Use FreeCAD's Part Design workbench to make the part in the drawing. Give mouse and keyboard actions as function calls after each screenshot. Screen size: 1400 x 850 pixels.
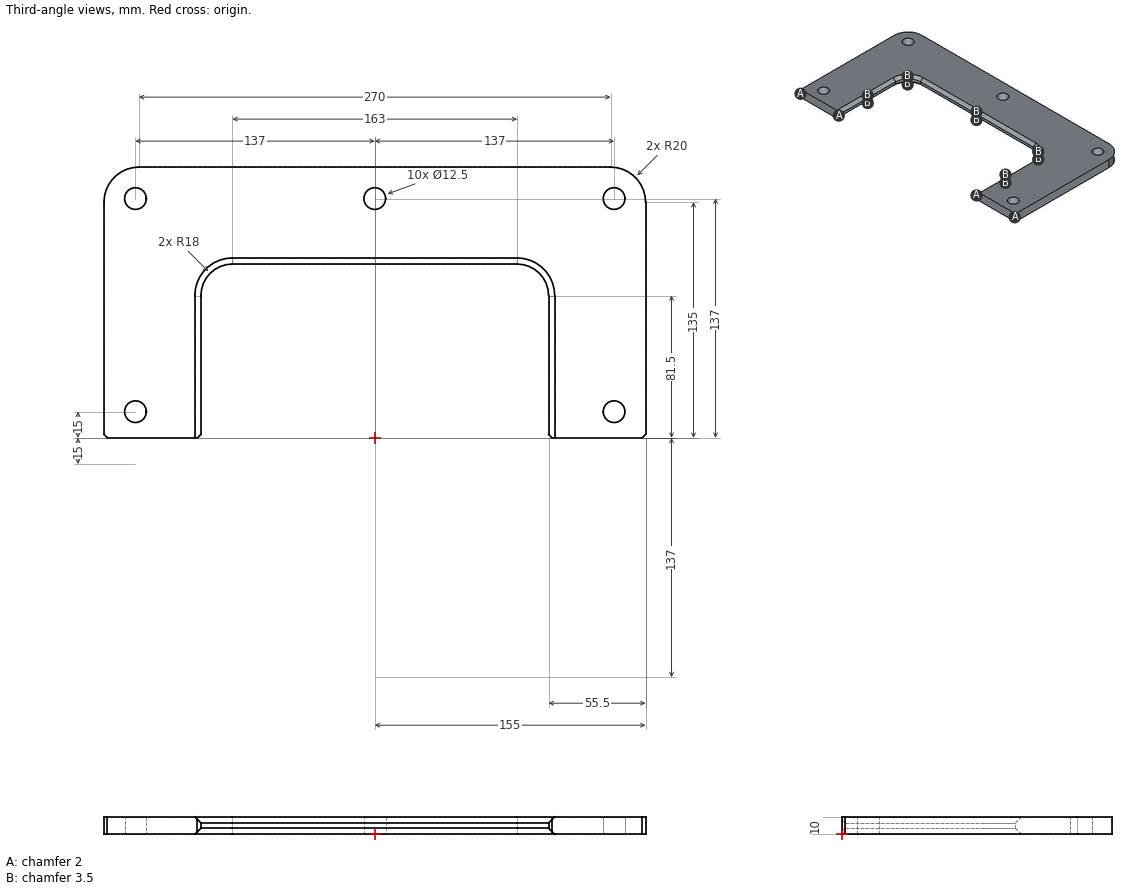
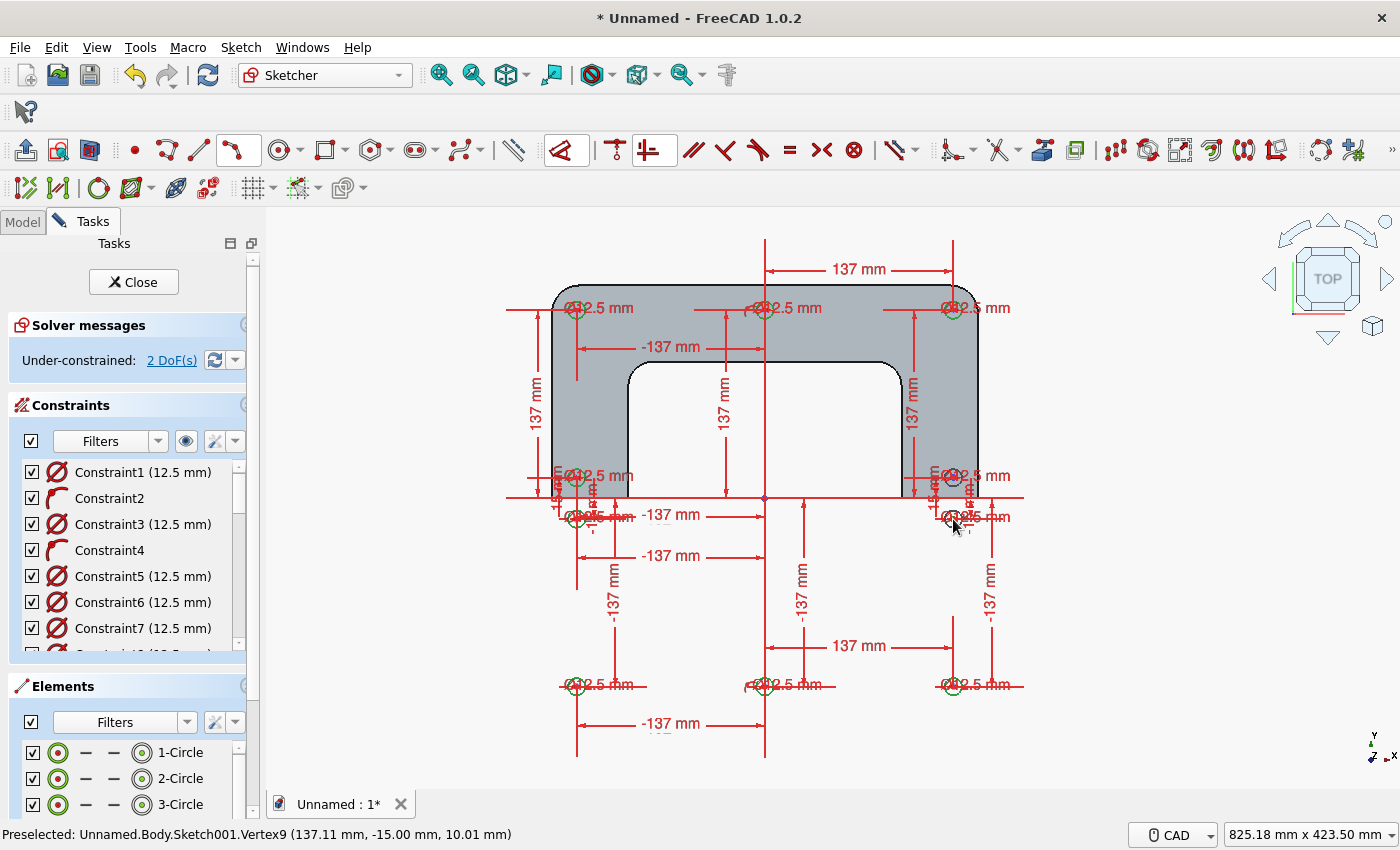
key(l)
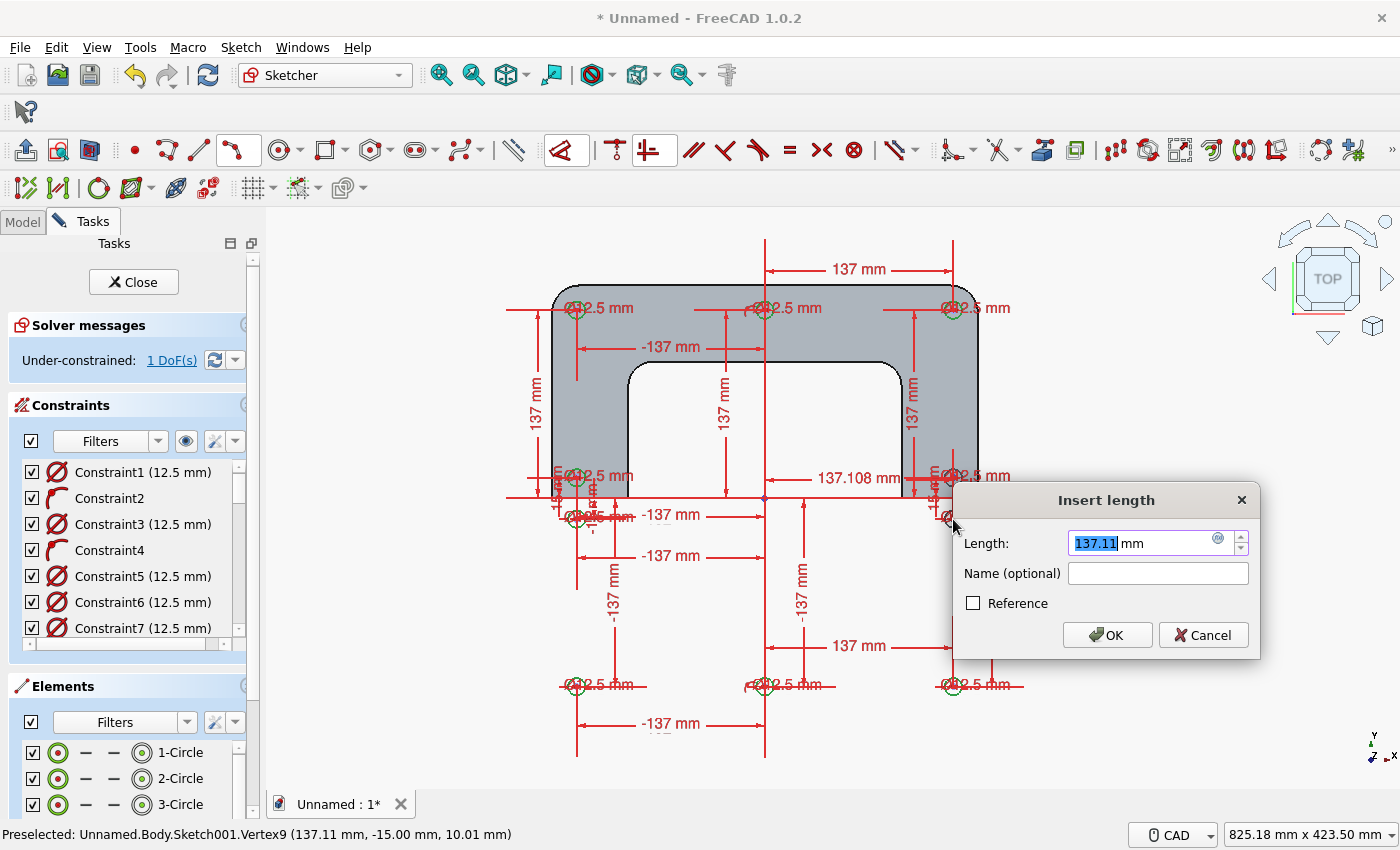
text(137)
key(Return)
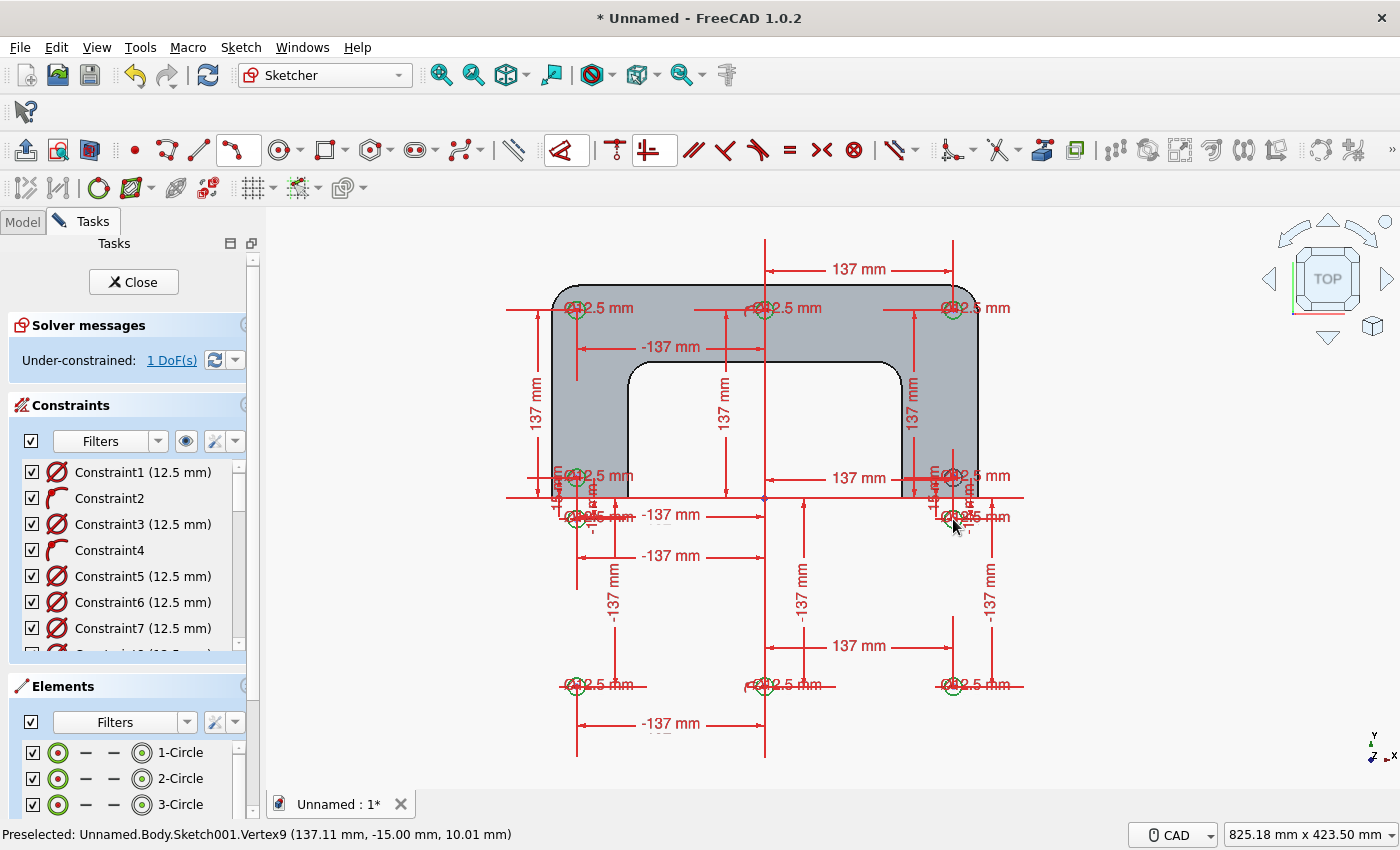
click(953, 478)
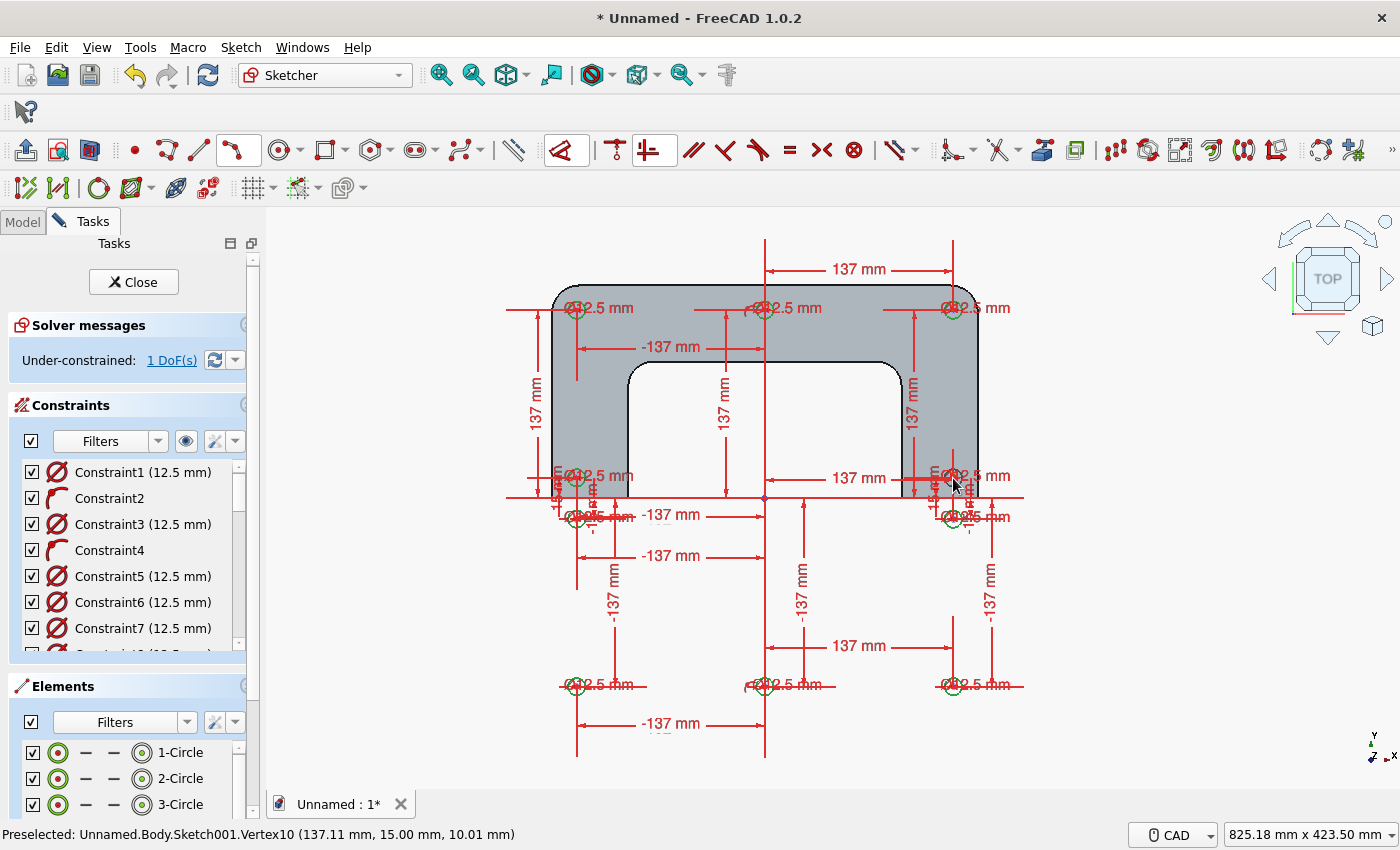
key(l)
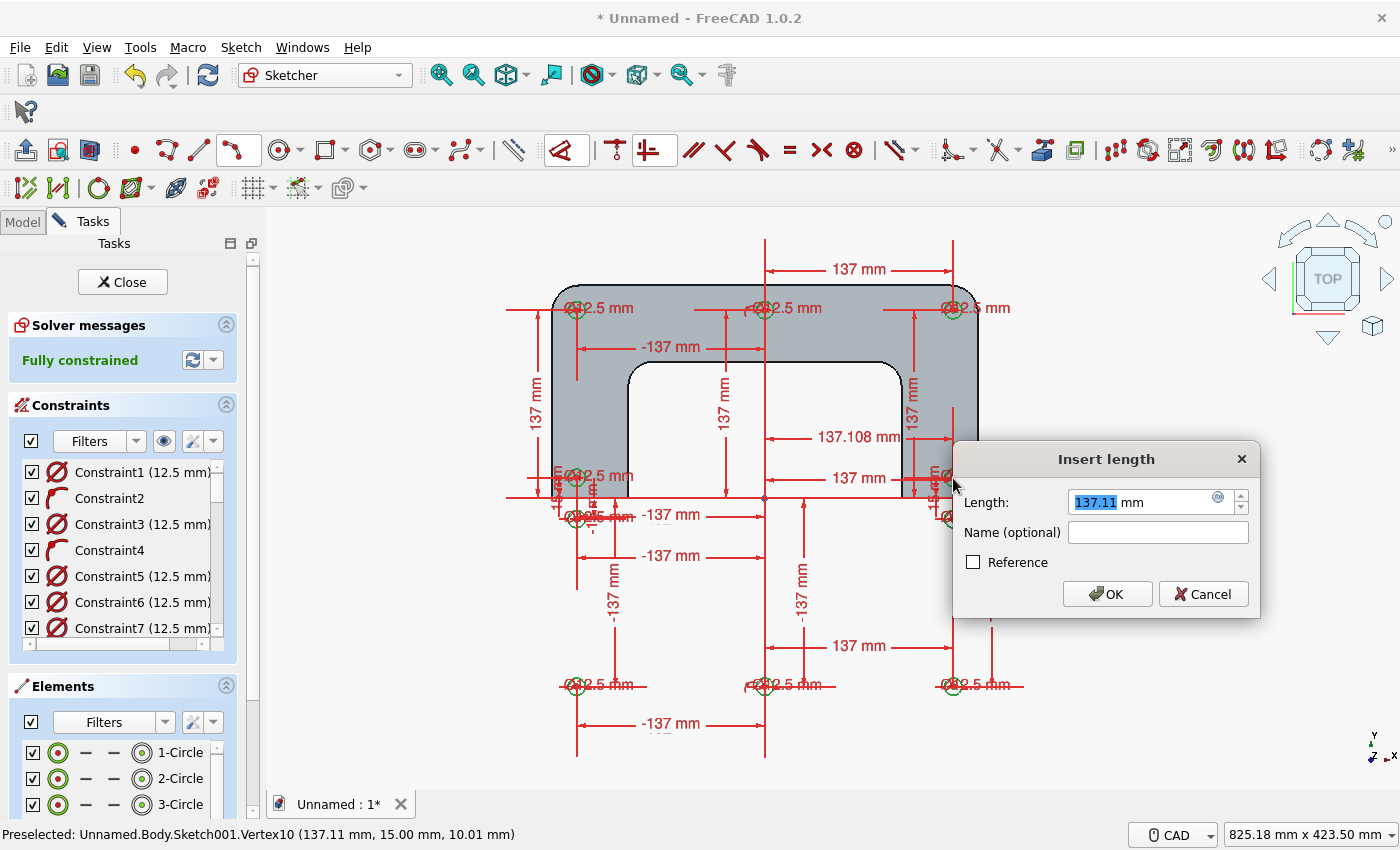
text(137)
key(Return)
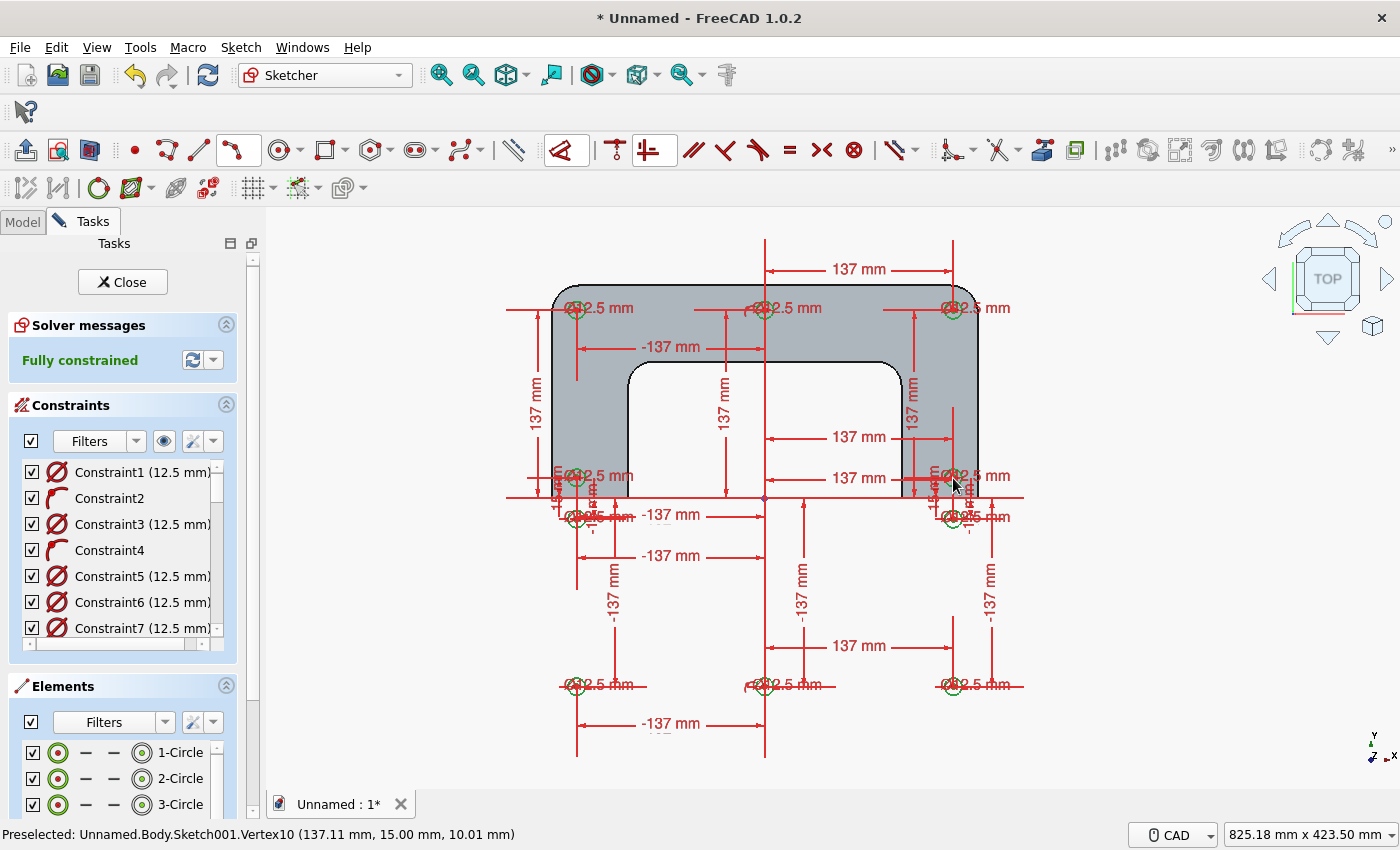
click(123, 282)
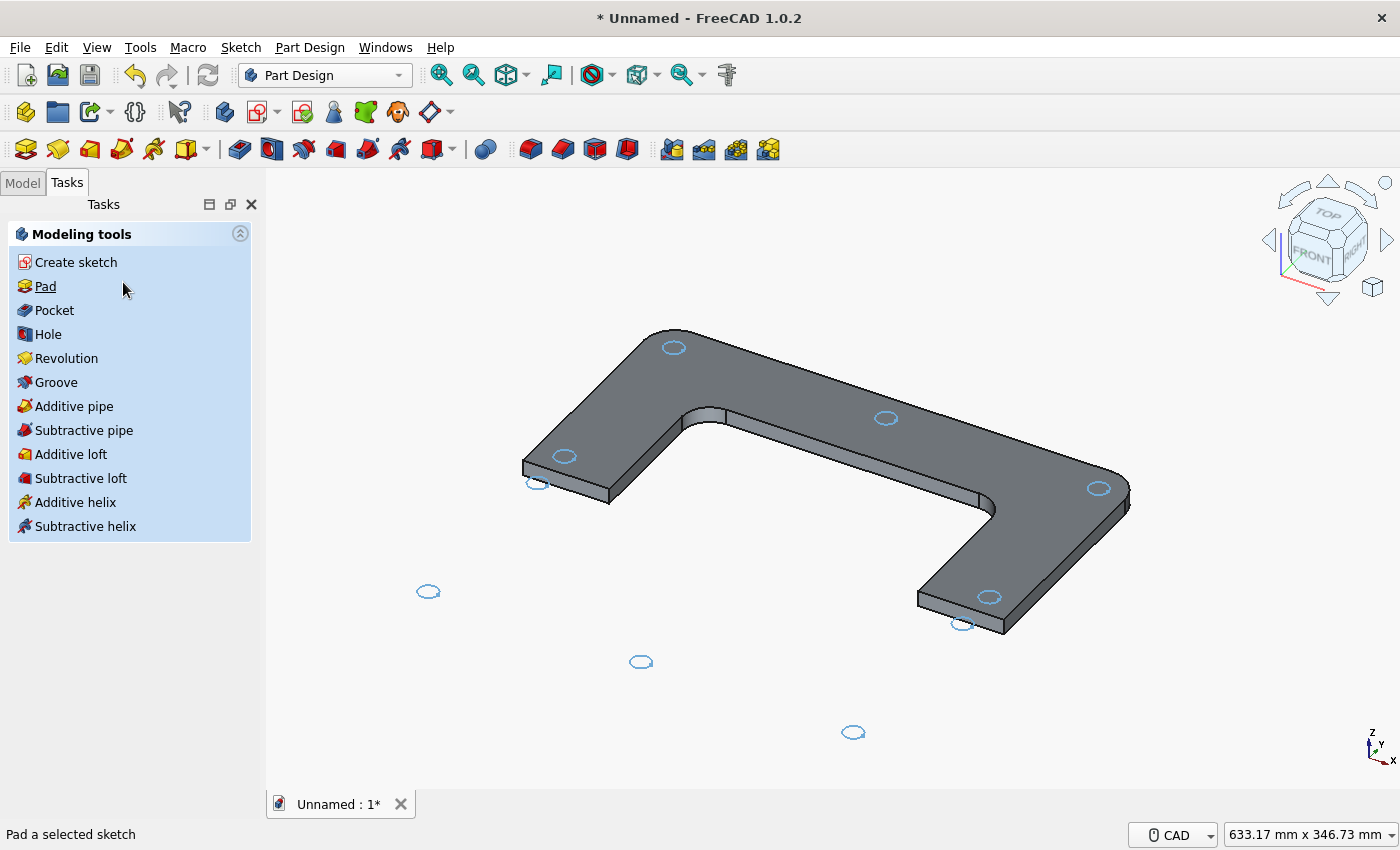
click(240, 150)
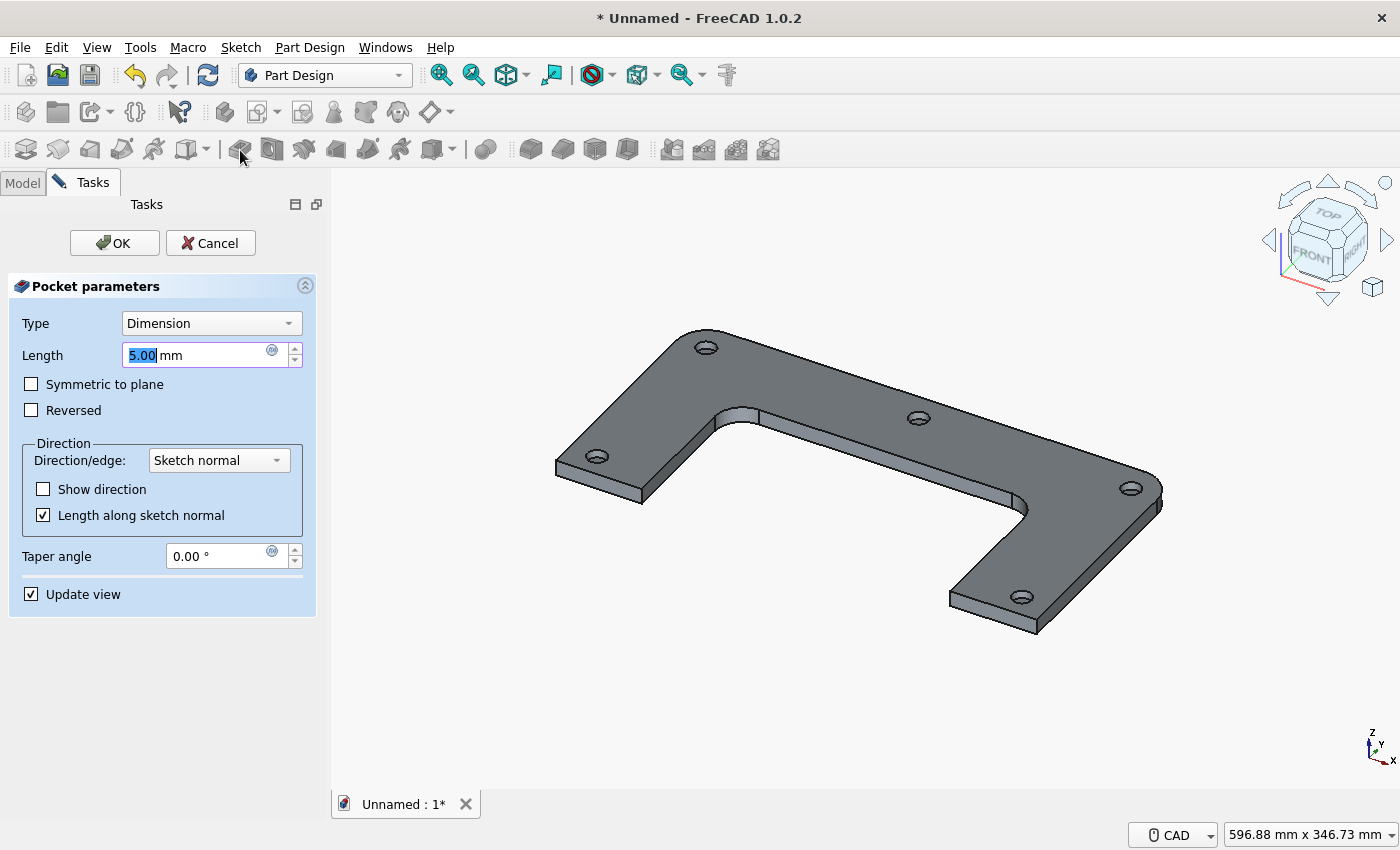
click(212, 324)